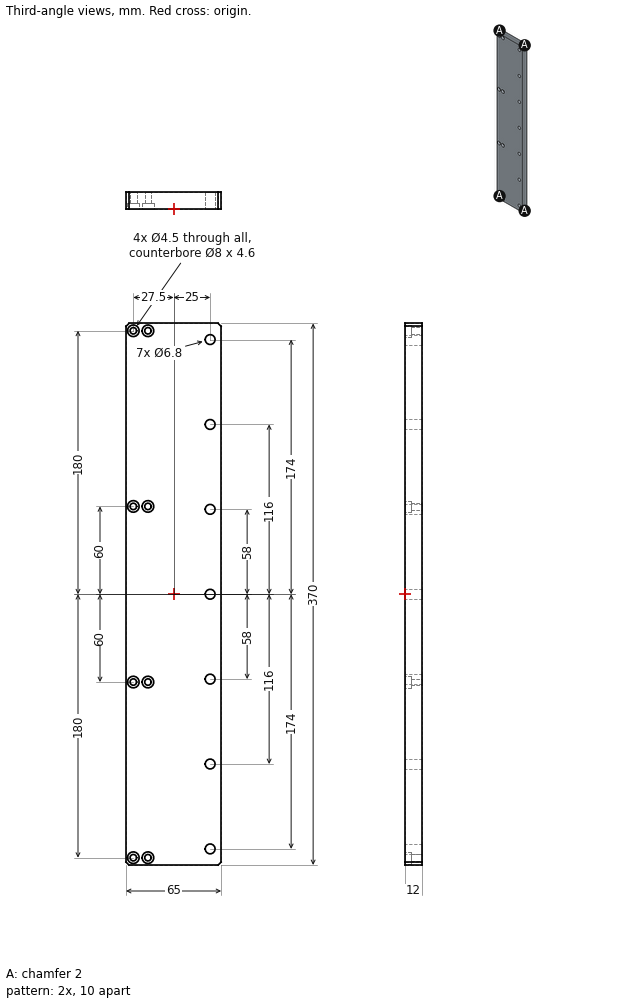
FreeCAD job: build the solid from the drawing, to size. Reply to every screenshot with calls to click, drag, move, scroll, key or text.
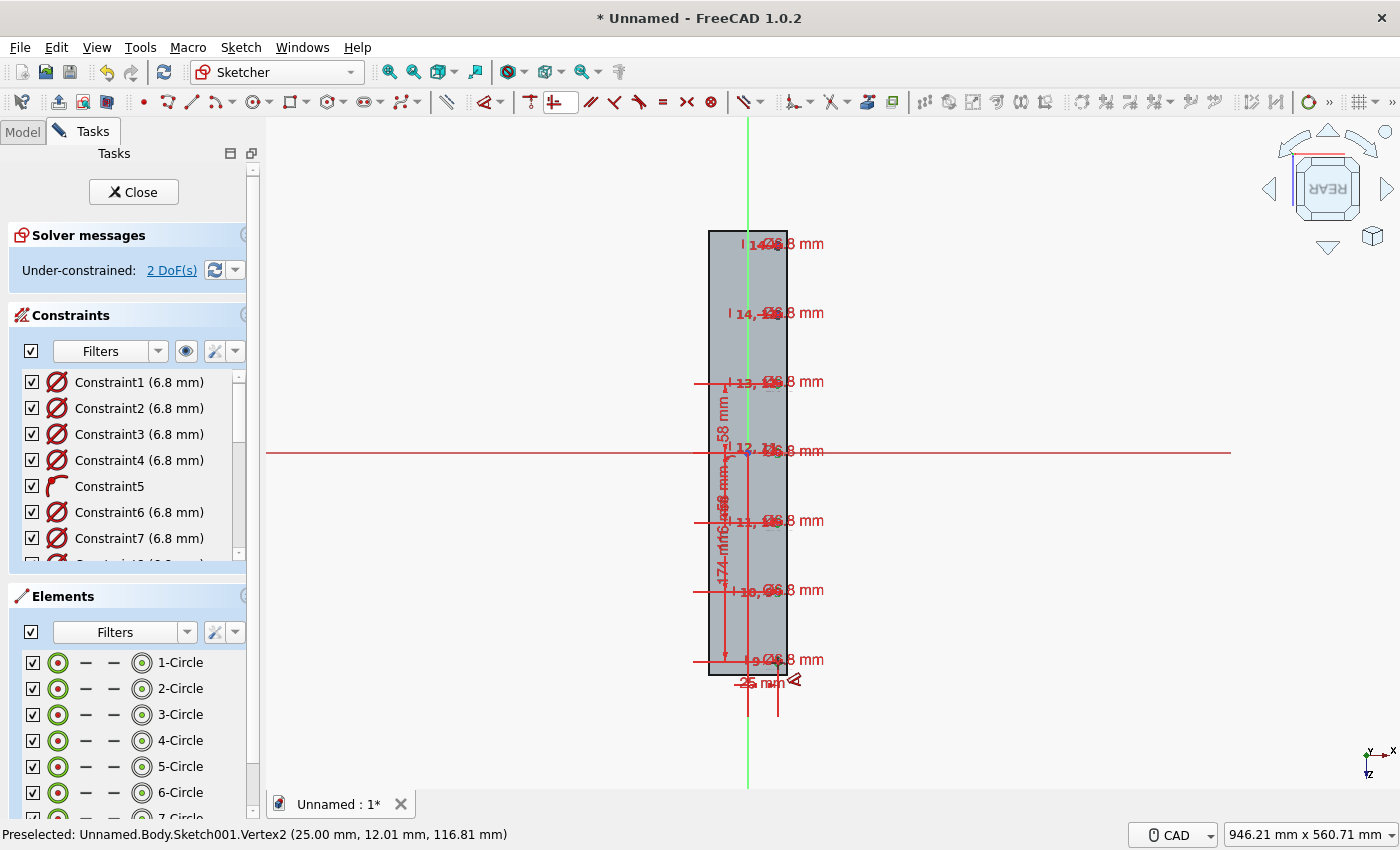
click(778, 315)
click(714, 384)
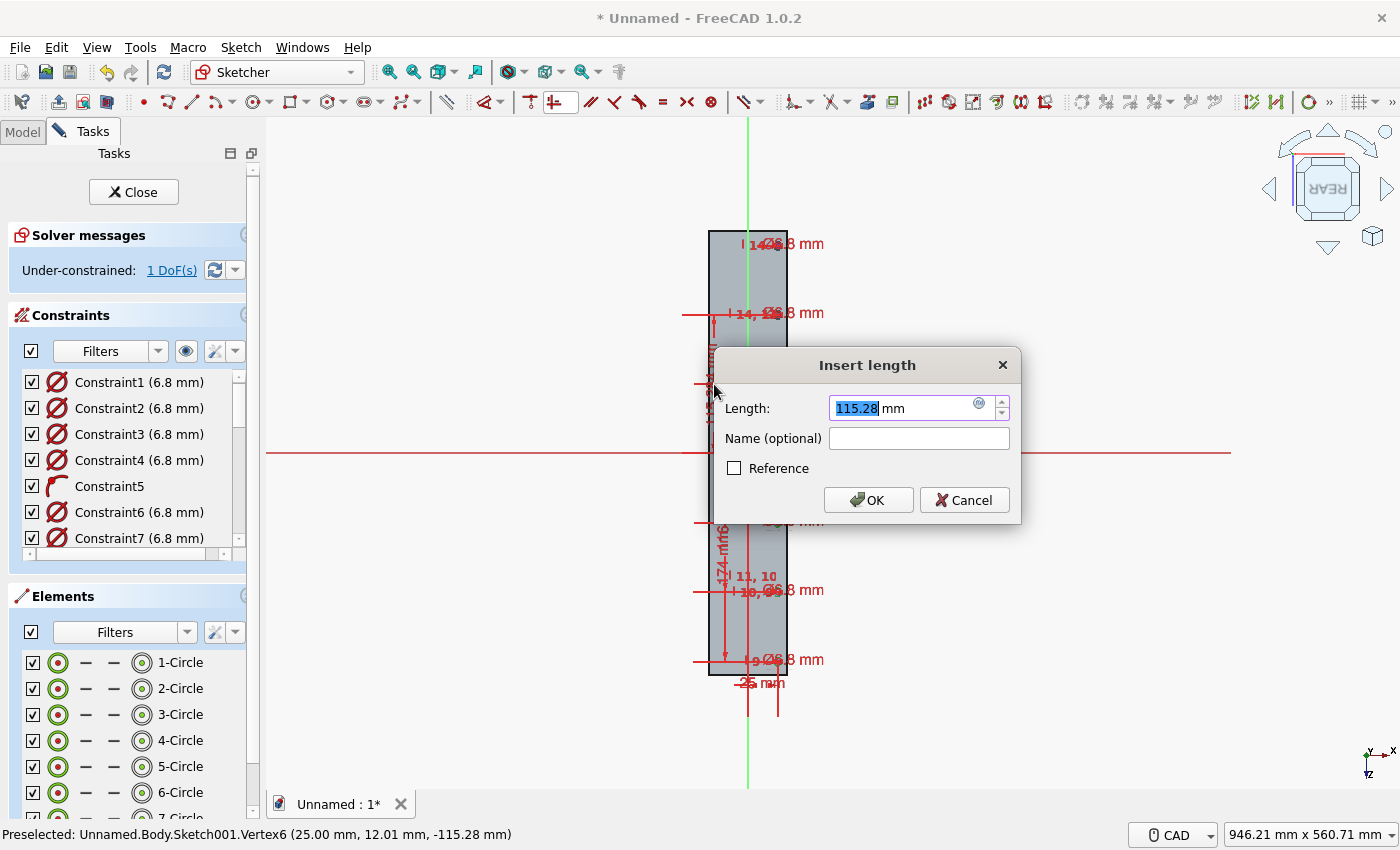
text(116)
key(Return)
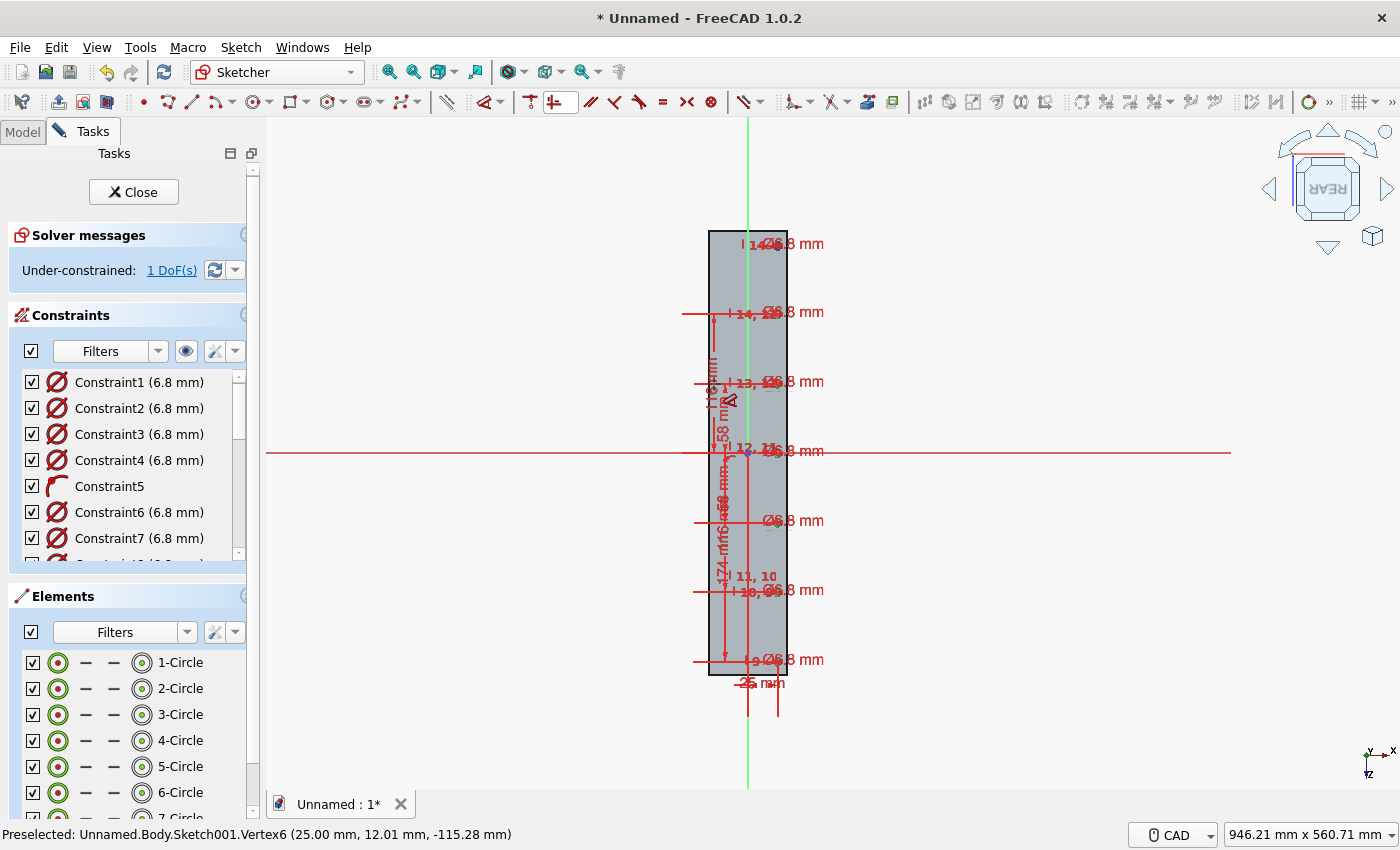
click(778, 246)
click(714, 350)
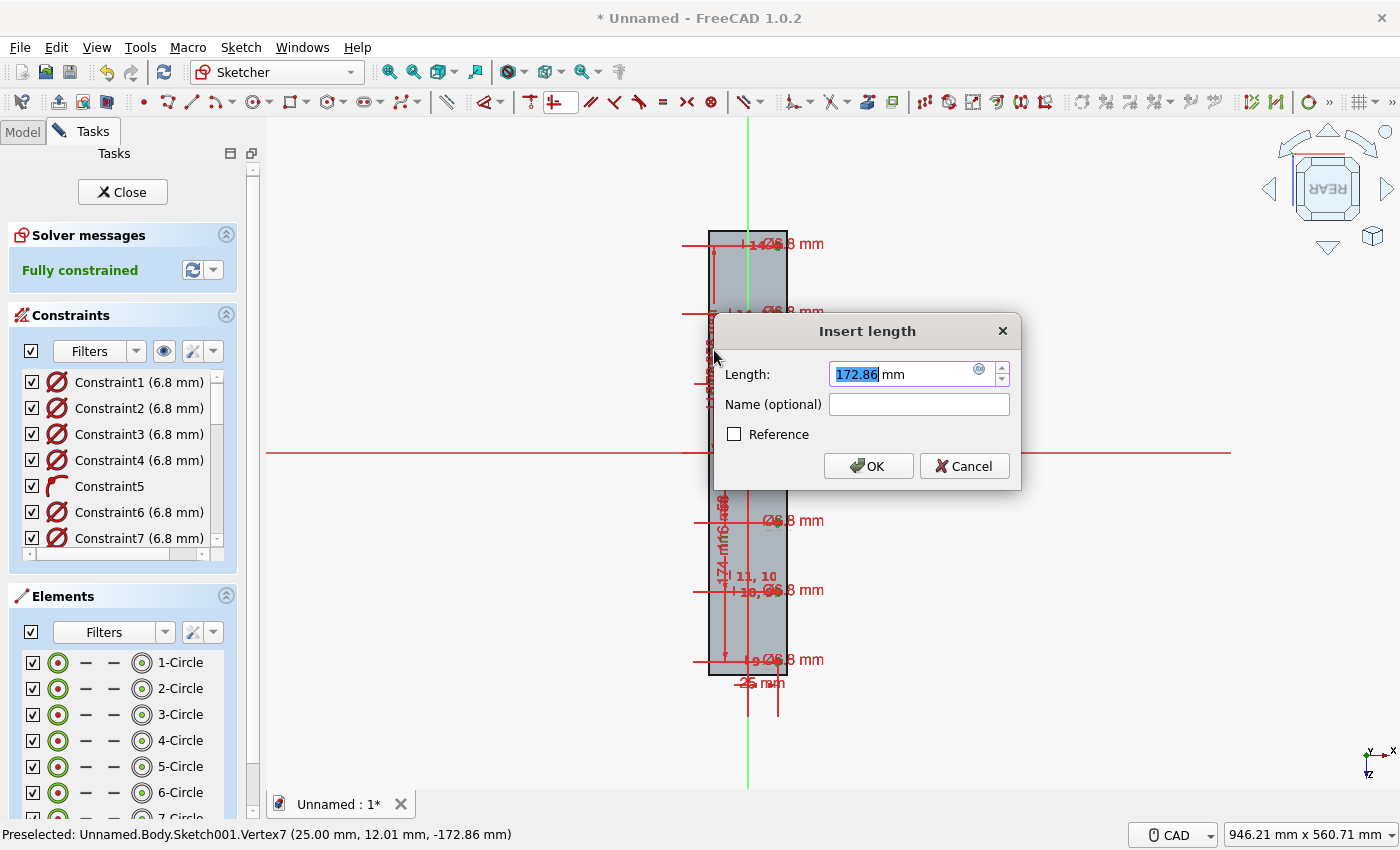
text(174)
key(Return)
key(Escape)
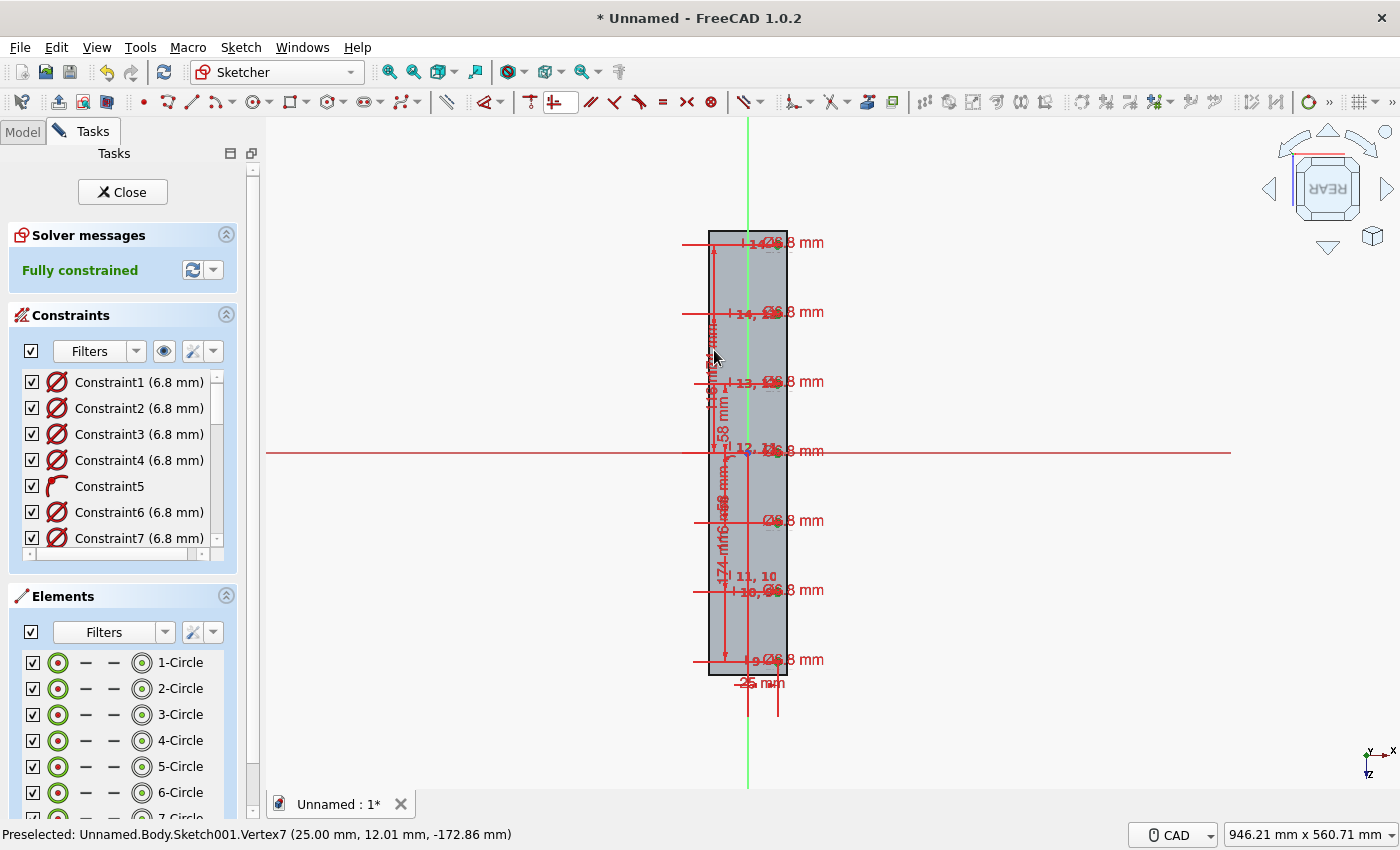
click(123, 192)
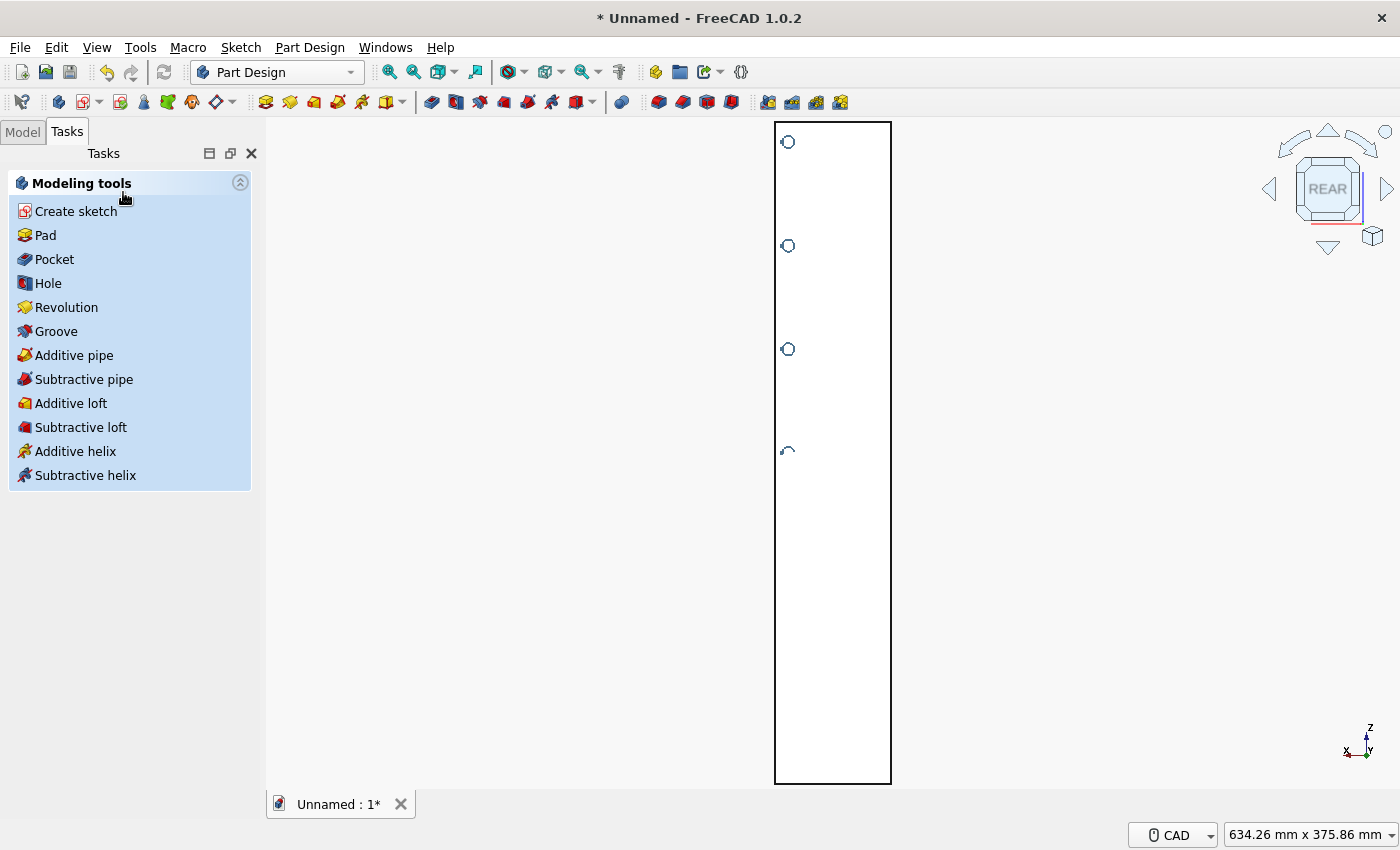
click(432, 102)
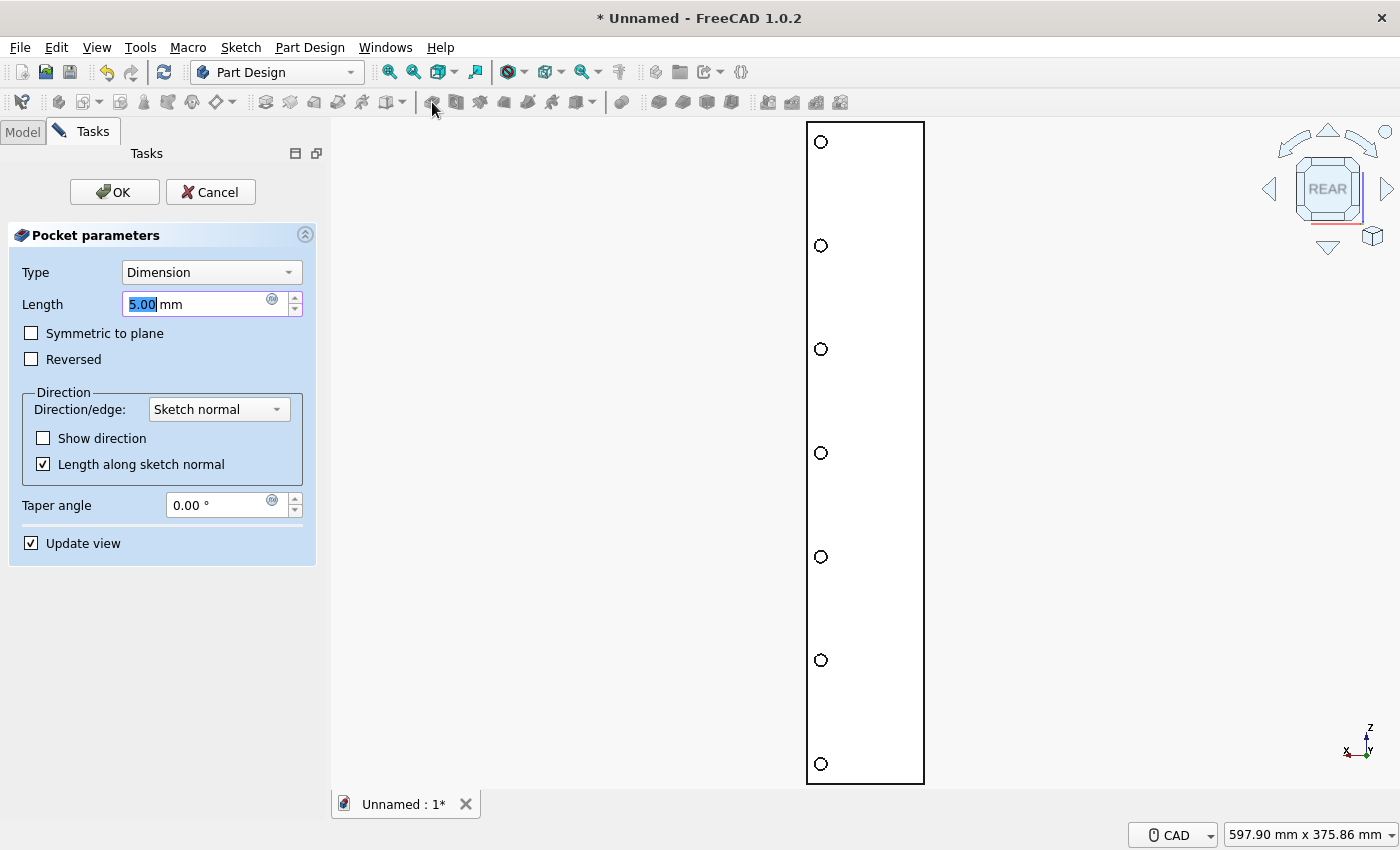
click(212, 272)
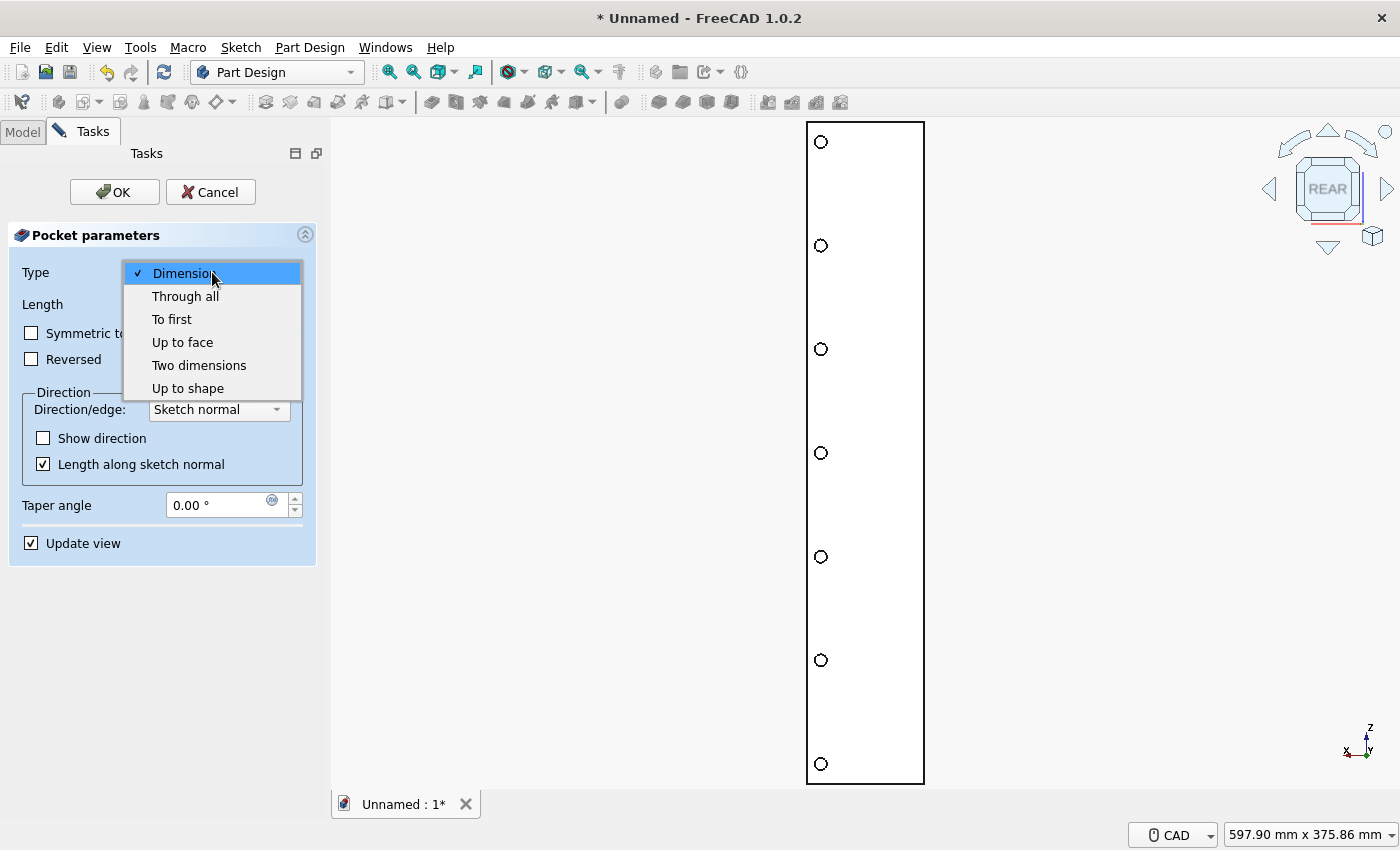
click(212, 296)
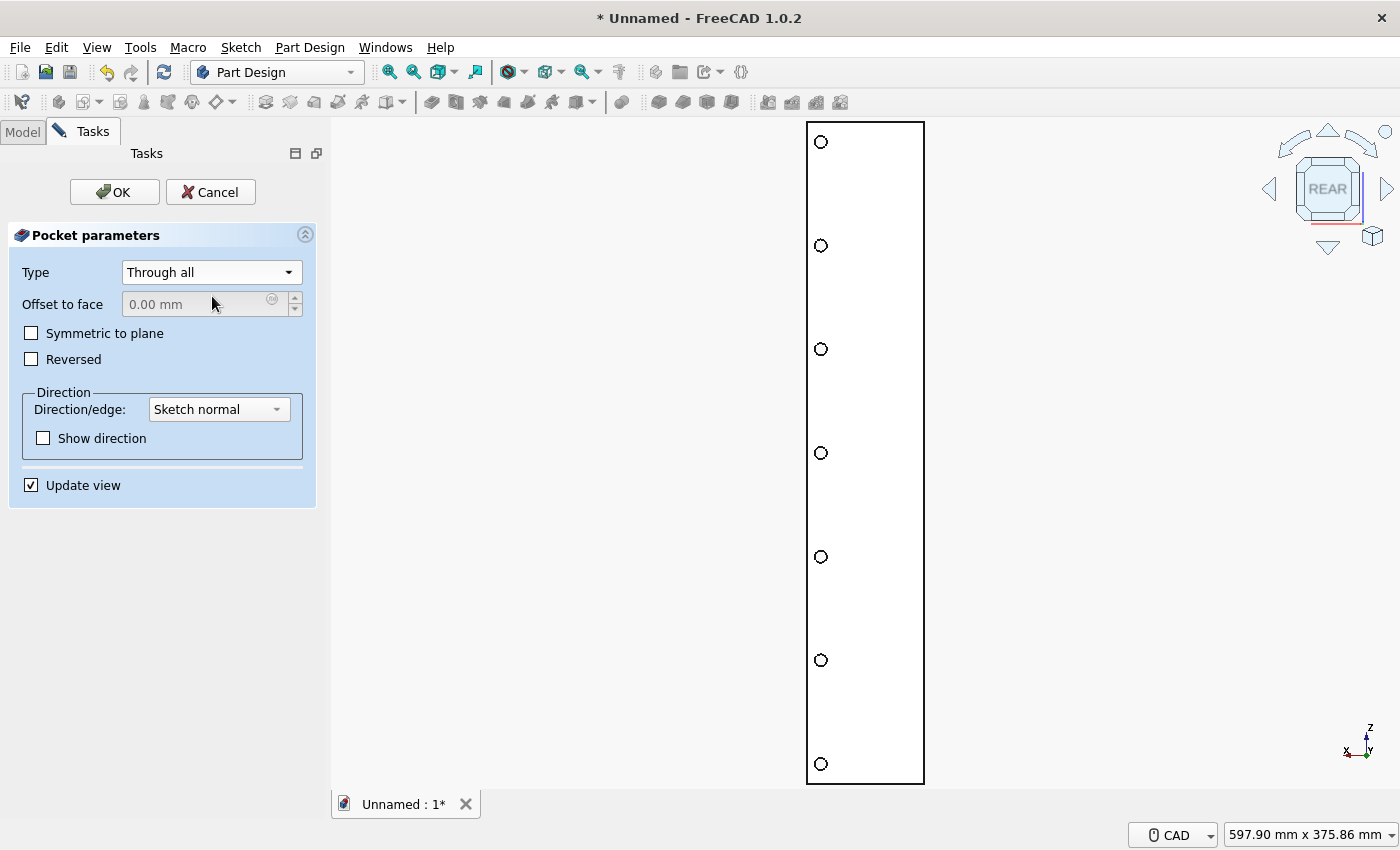
click(115, 192)